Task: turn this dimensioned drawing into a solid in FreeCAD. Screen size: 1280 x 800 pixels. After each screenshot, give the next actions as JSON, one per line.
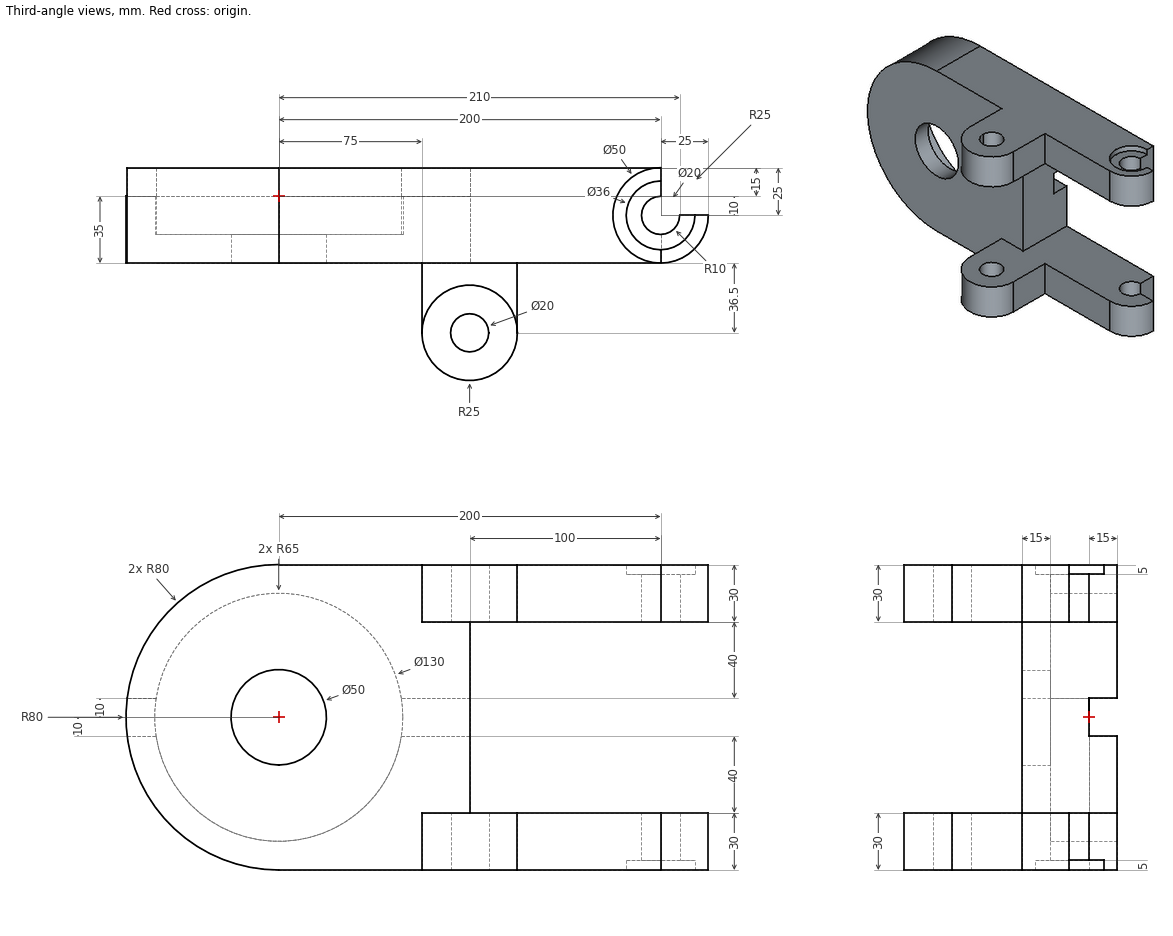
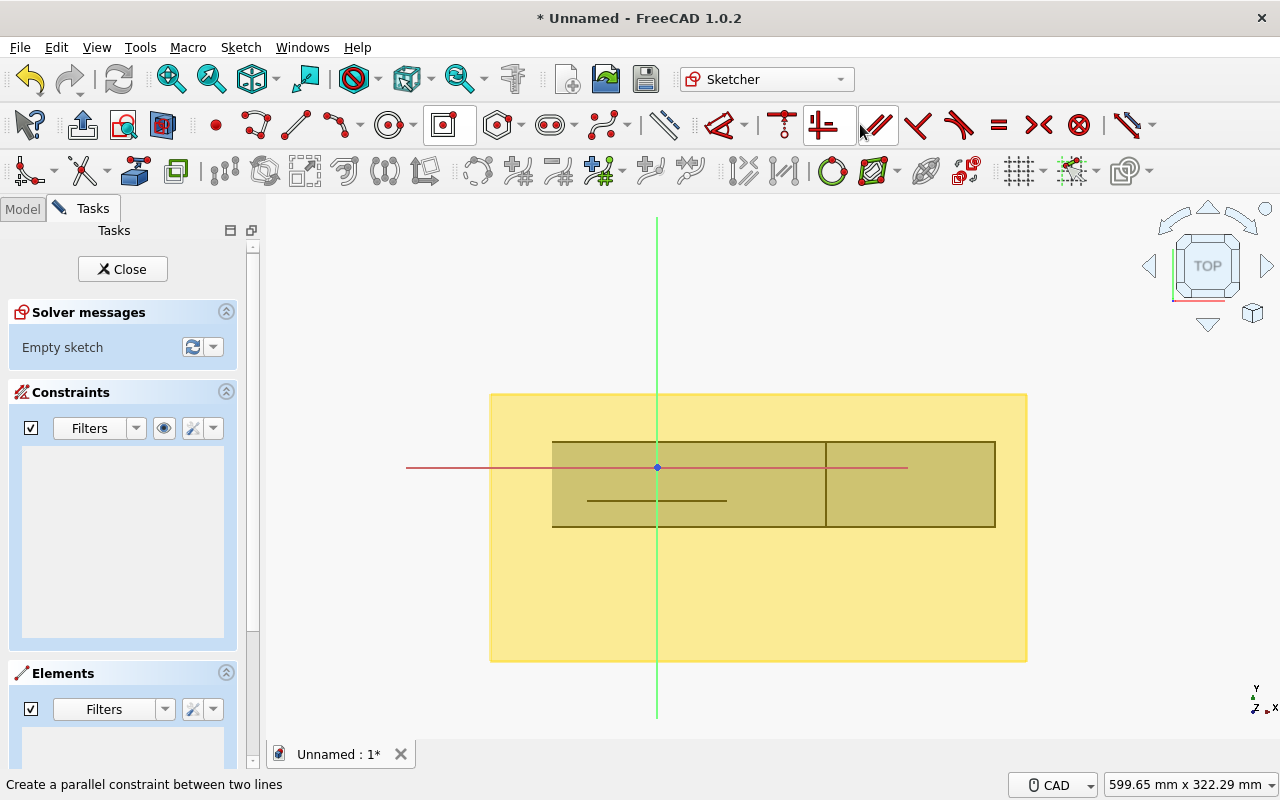
{"action": "scroll", "coordinate": [811, 617], "scroll_direction": "up", "scroll_amount": 4}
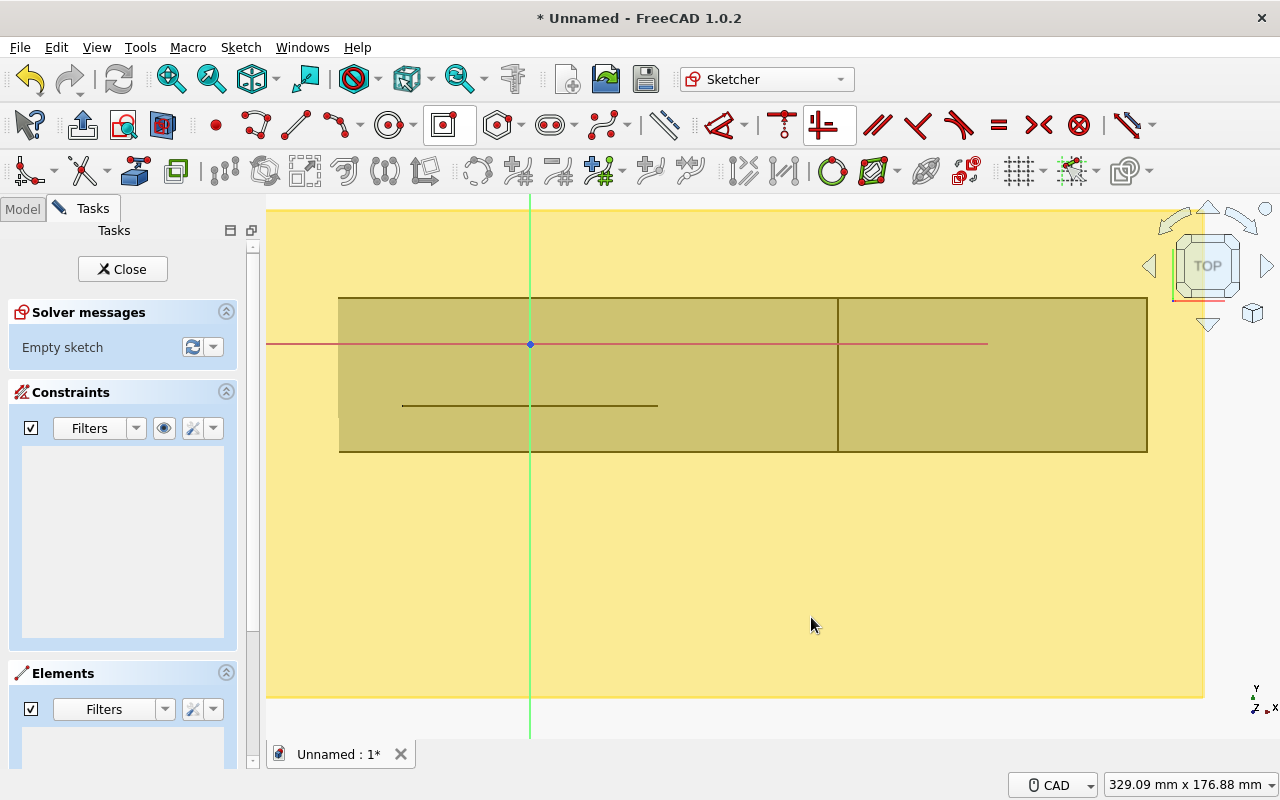
{"action": "left_click", "coordinate": [256, 126]}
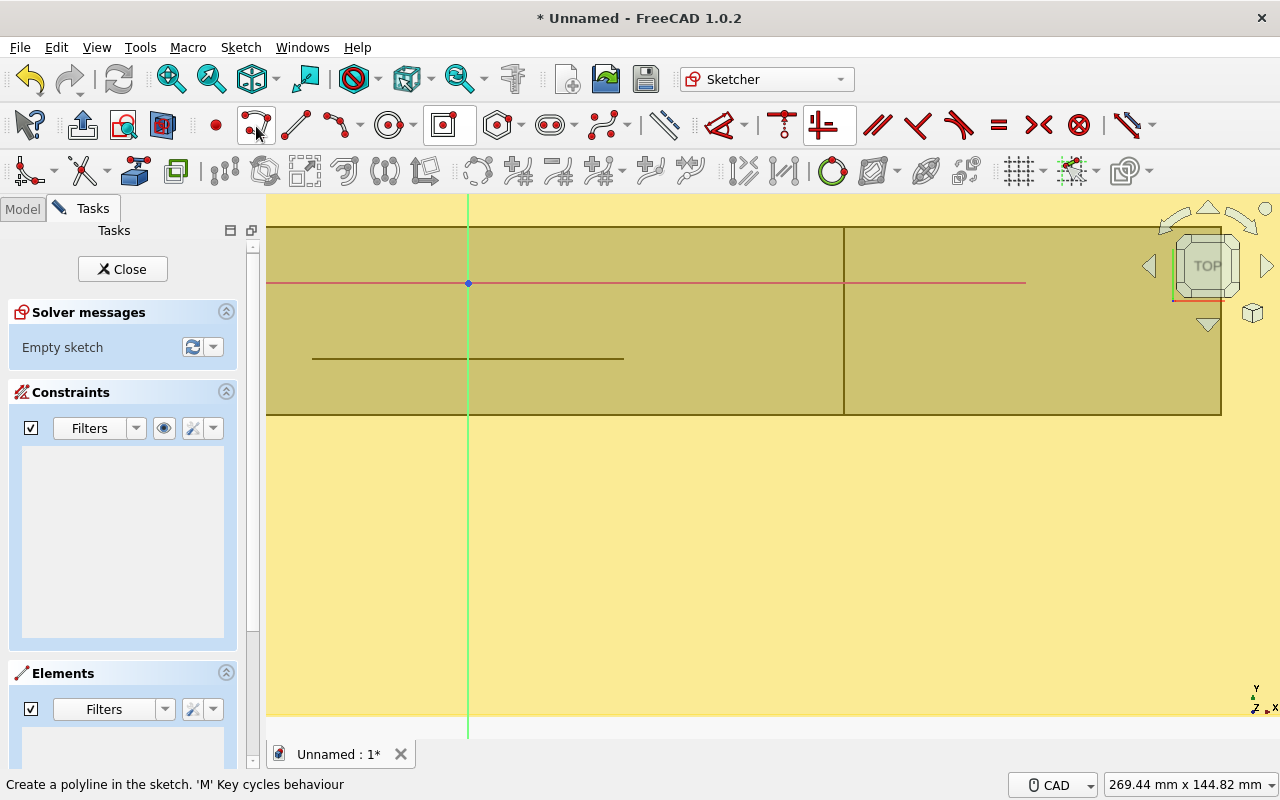
{"action": "left_click", "coordinate": [750, 553]}
{"action": "left_click", "coordinate": [750, 415]}
{"action": "left_click", "coordinate": [938, 415]}
{"action": "left_click", "coordinate": [938, 553]}
{"action": "right_click", "coordinate": [938, 553]}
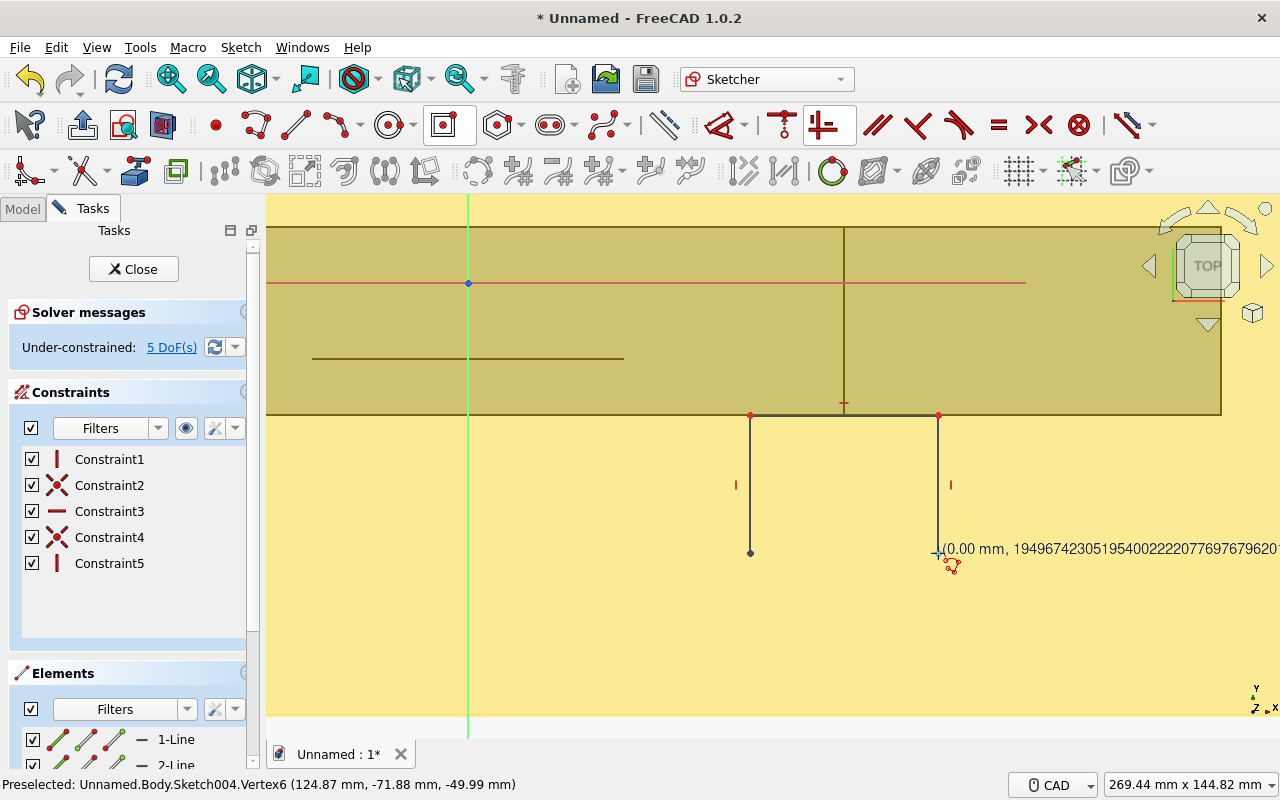
{"action": "key", "text": "g 3 a"}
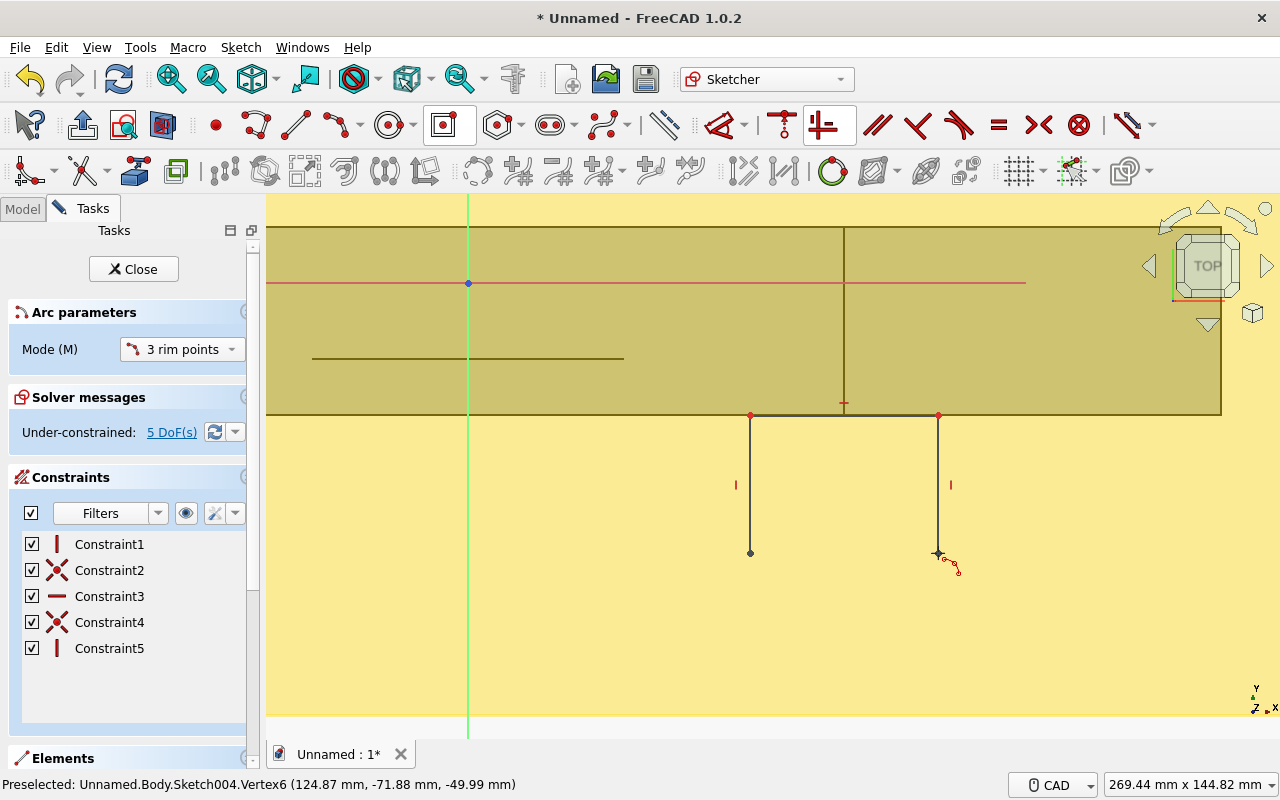
{"action": "left_click", "coordinate": [938, 554]}
{"action": "left_click", "coordinate": [750, 554]}
{"action": "left_click", "coordinate": [844, 647]}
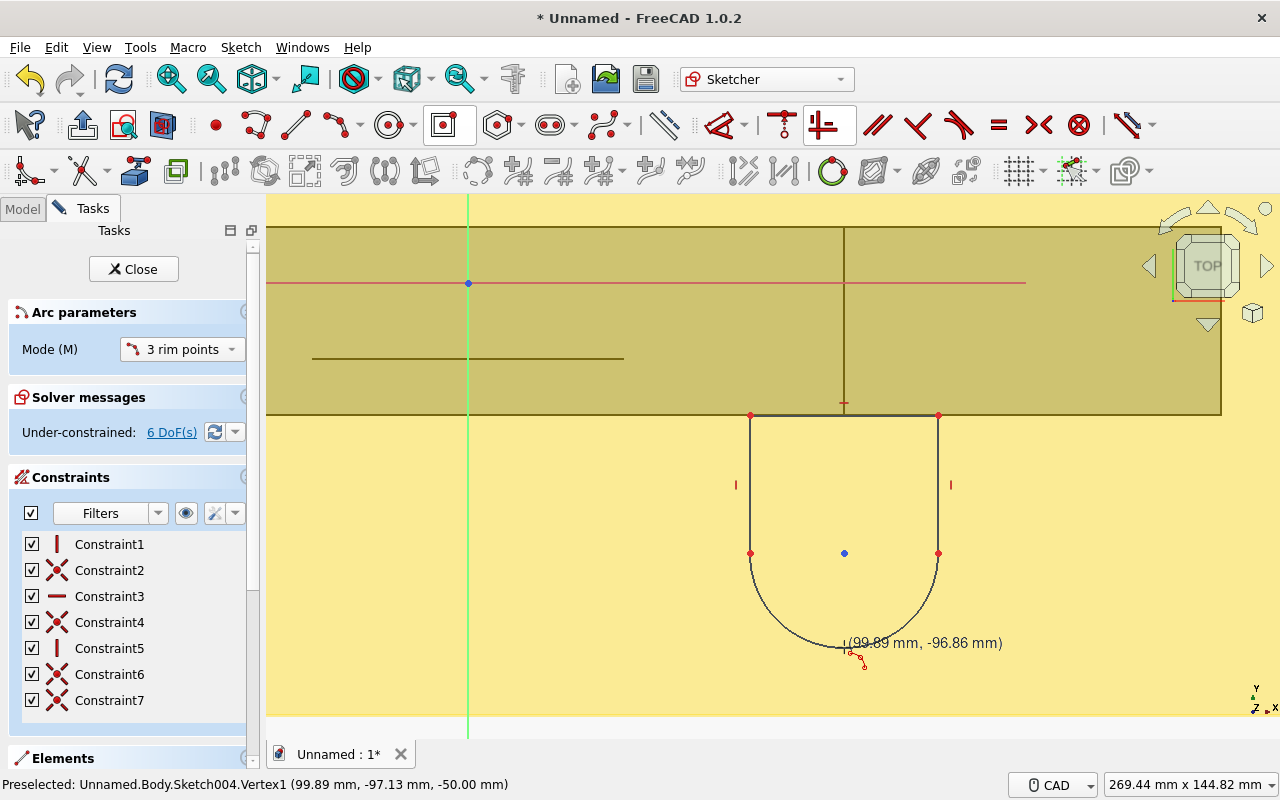
{"action": "left_click", "coordinate": [390, 126]}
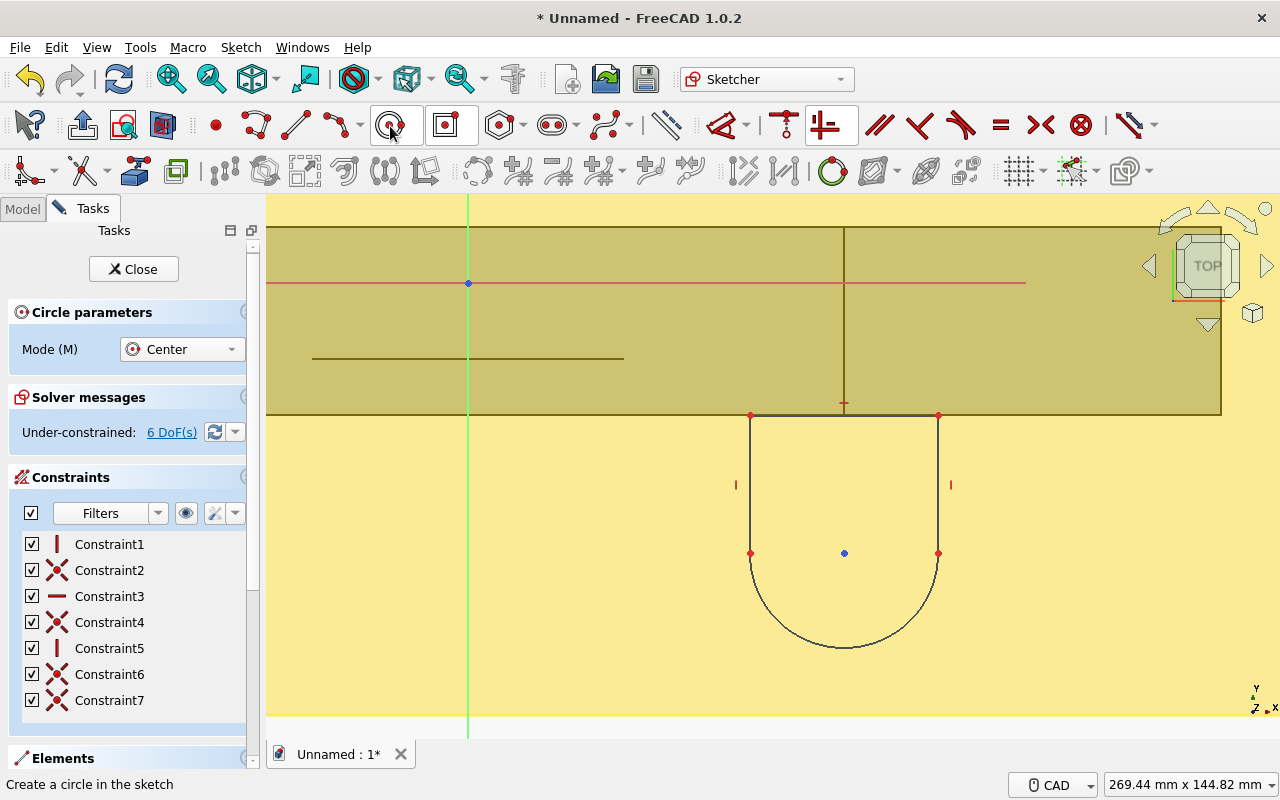
{"action": "left_click", "coordinate": [844, 553]}
{"action": "left_click", "coordinate": [871, 526]}
{"action": "key", "text": "Escape"}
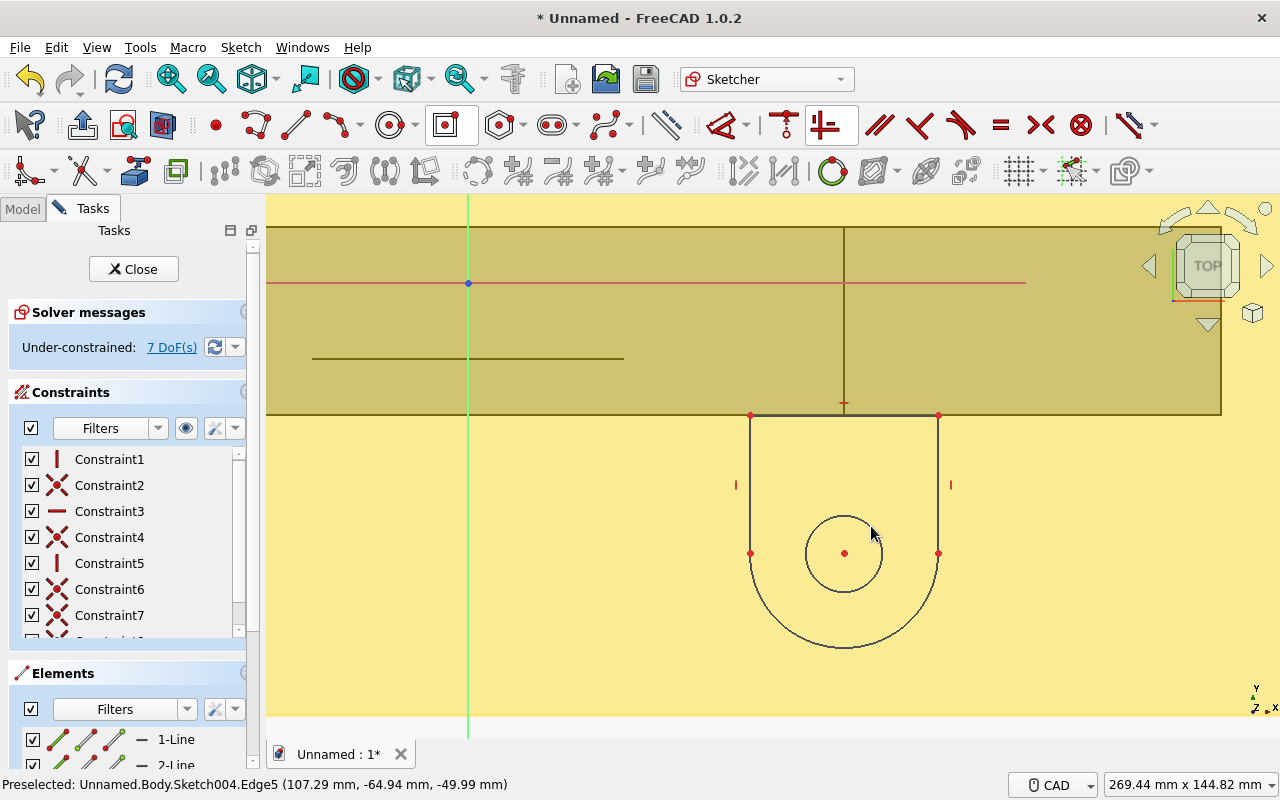
{"action": "left_click", "coordinate": [750, 513]}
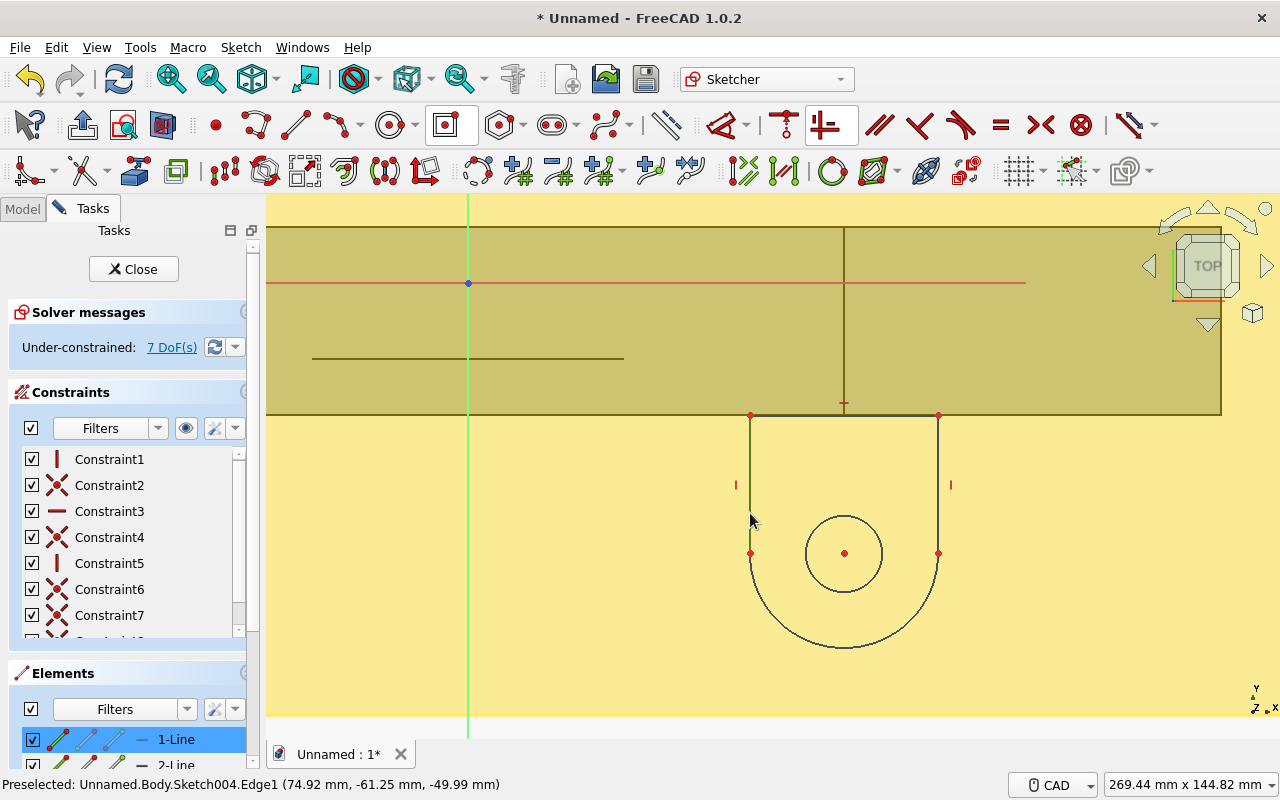
{"action": "left_click", "coordinate": [789, 630]}